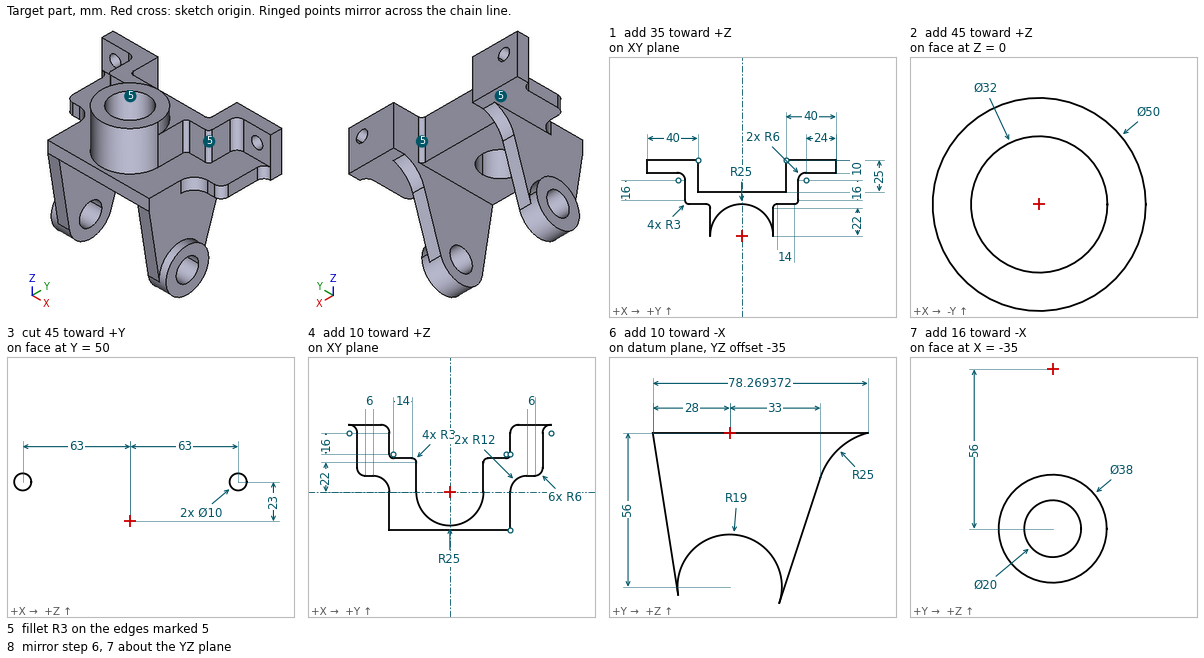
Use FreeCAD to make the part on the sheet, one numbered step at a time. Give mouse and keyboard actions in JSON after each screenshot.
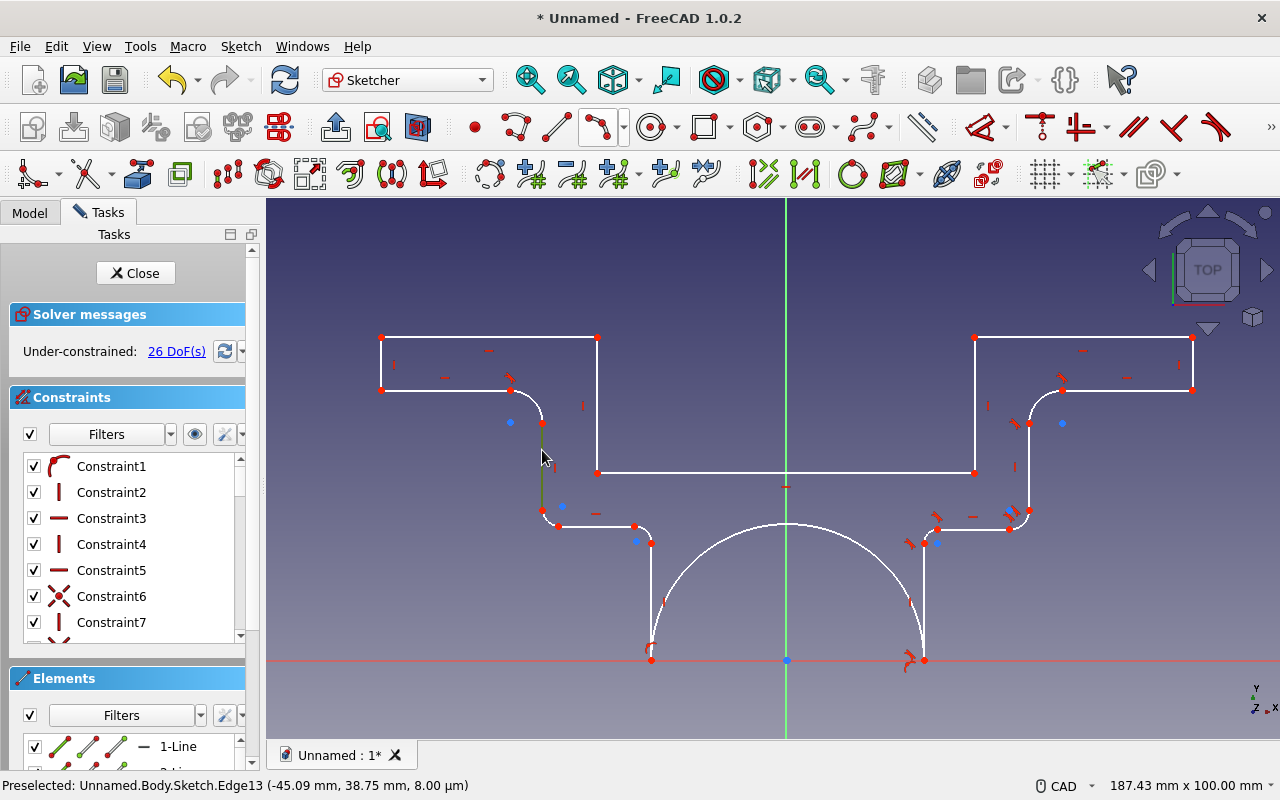
{"action": "left_click", "coordinate": [539, 409]}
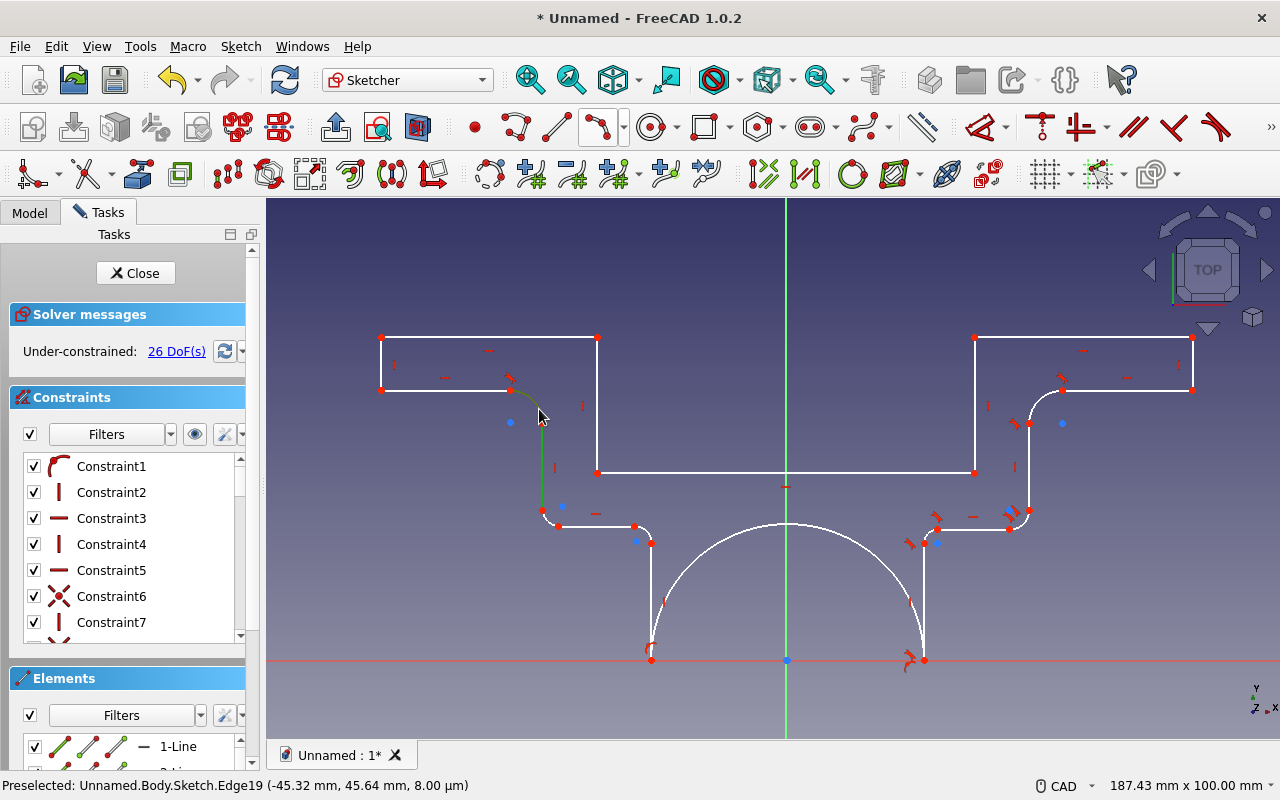
{"action": "left_click", "coordinate": [1216, 128]}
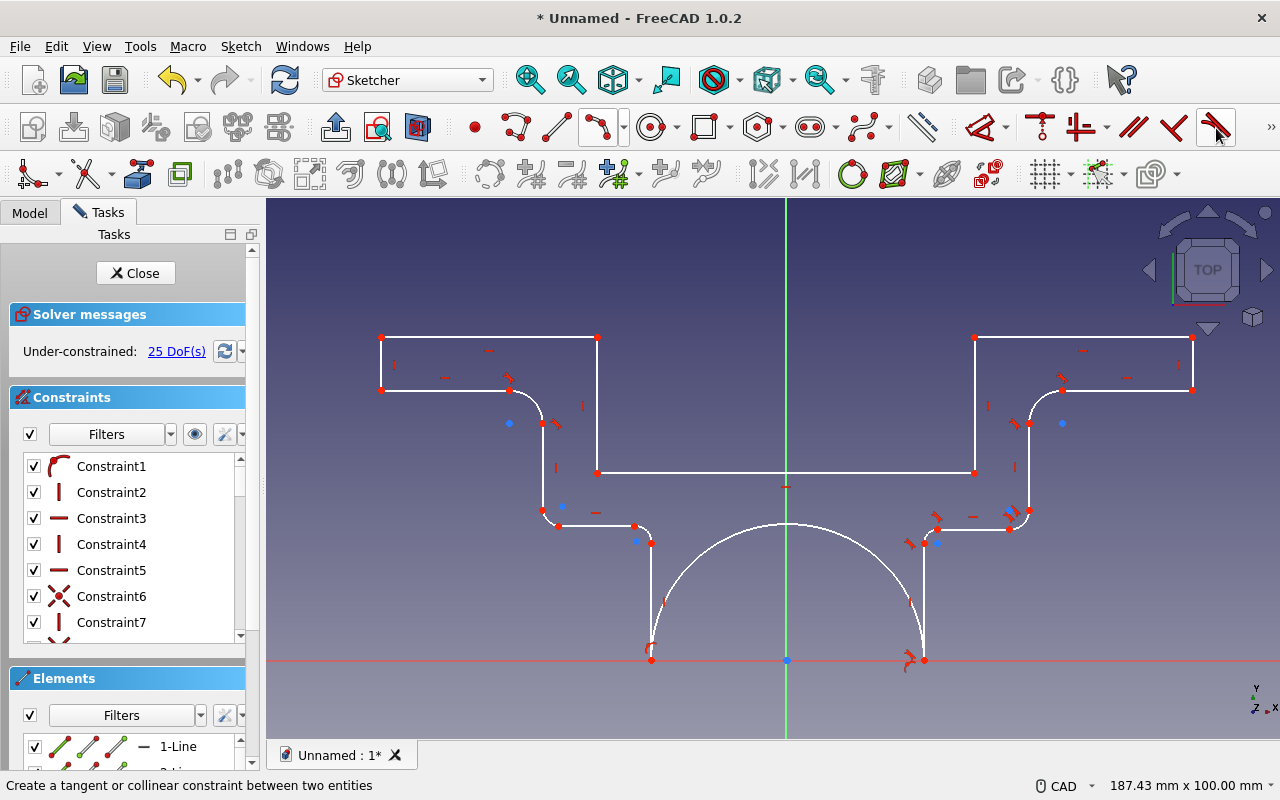
{"action": "left_click", "coordinate": [543, 450]}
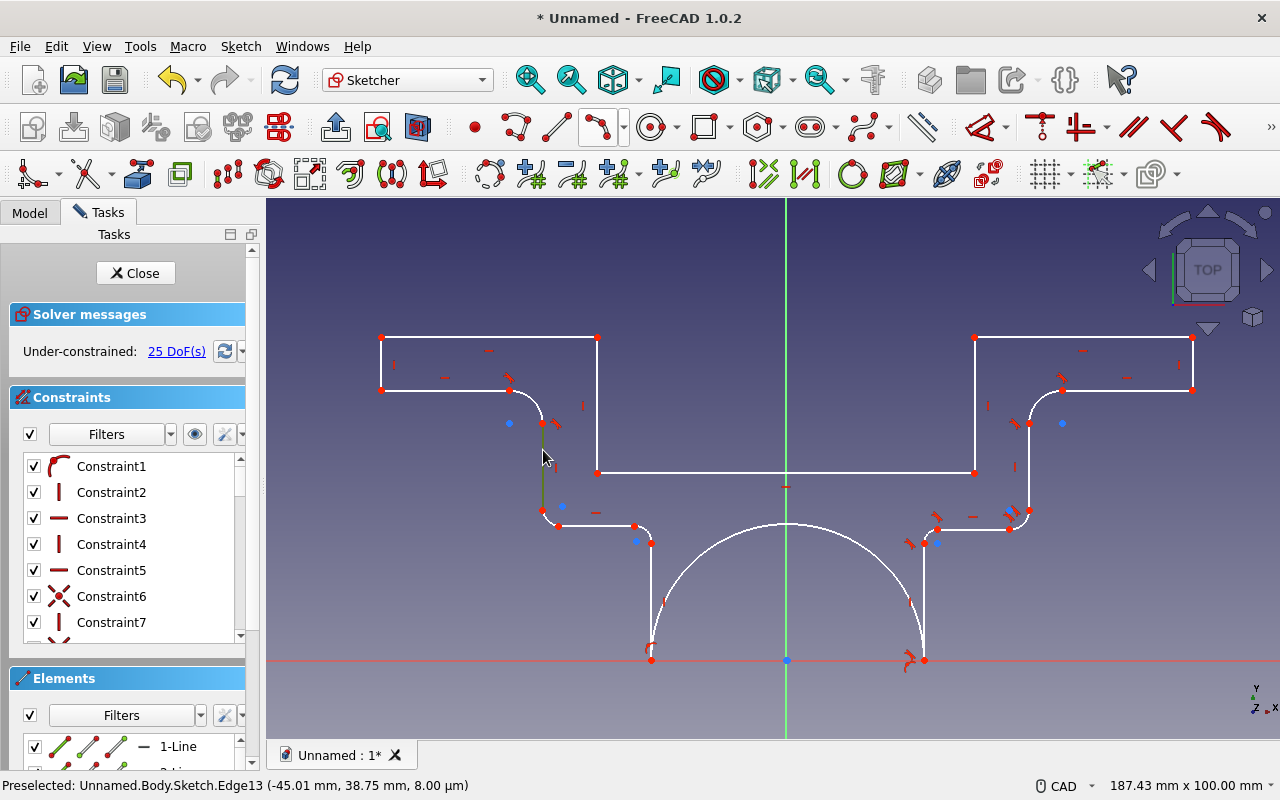
{"action": "left_click", "coordinate": [548, 521]}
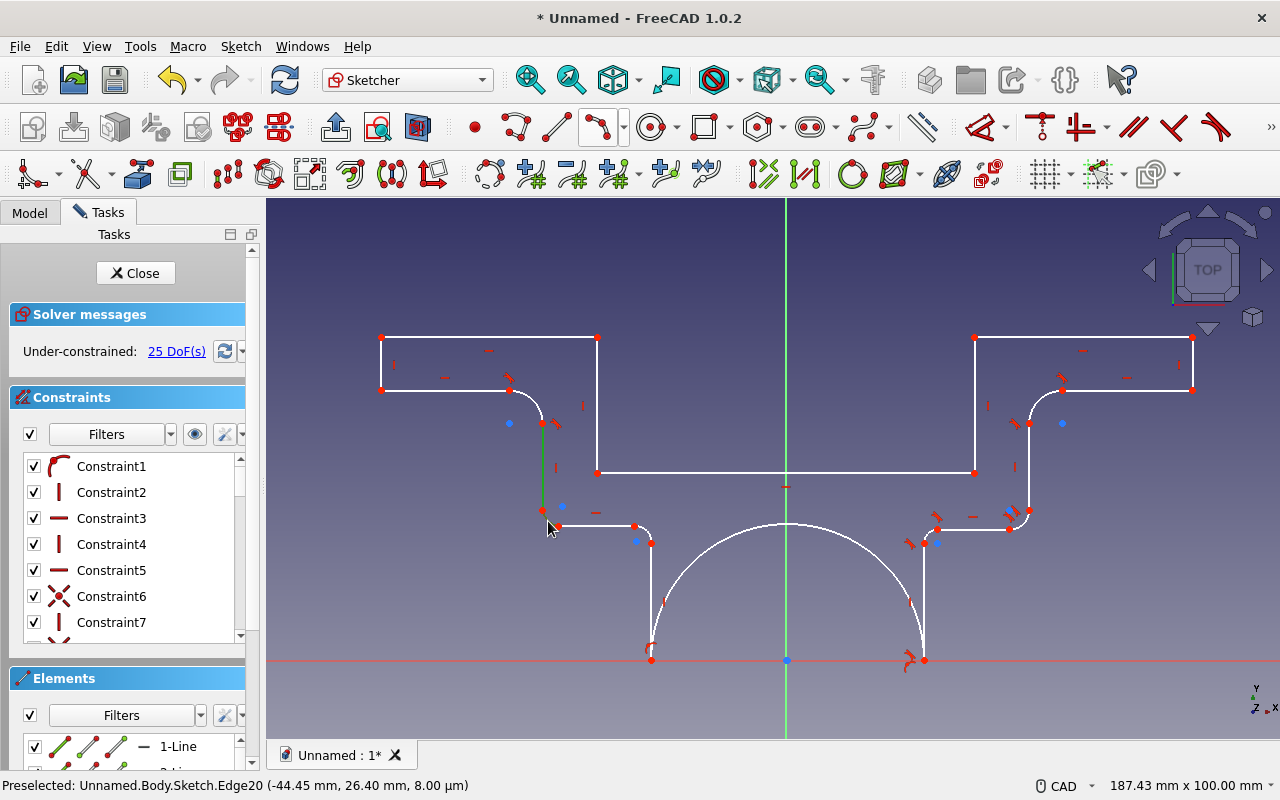
{"action": "left_click", "coordinate": [1216, 128]}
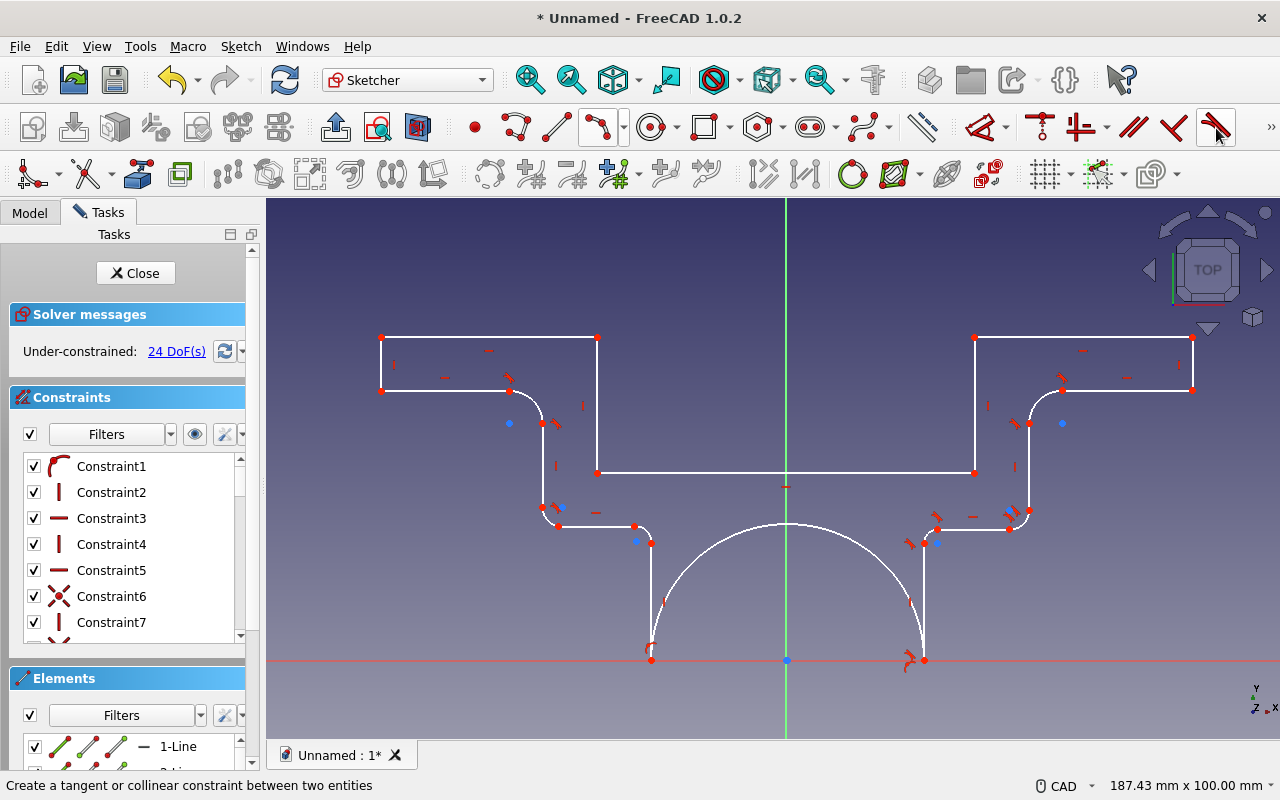
{"action": "left_click", "coordinate": [582, 527]}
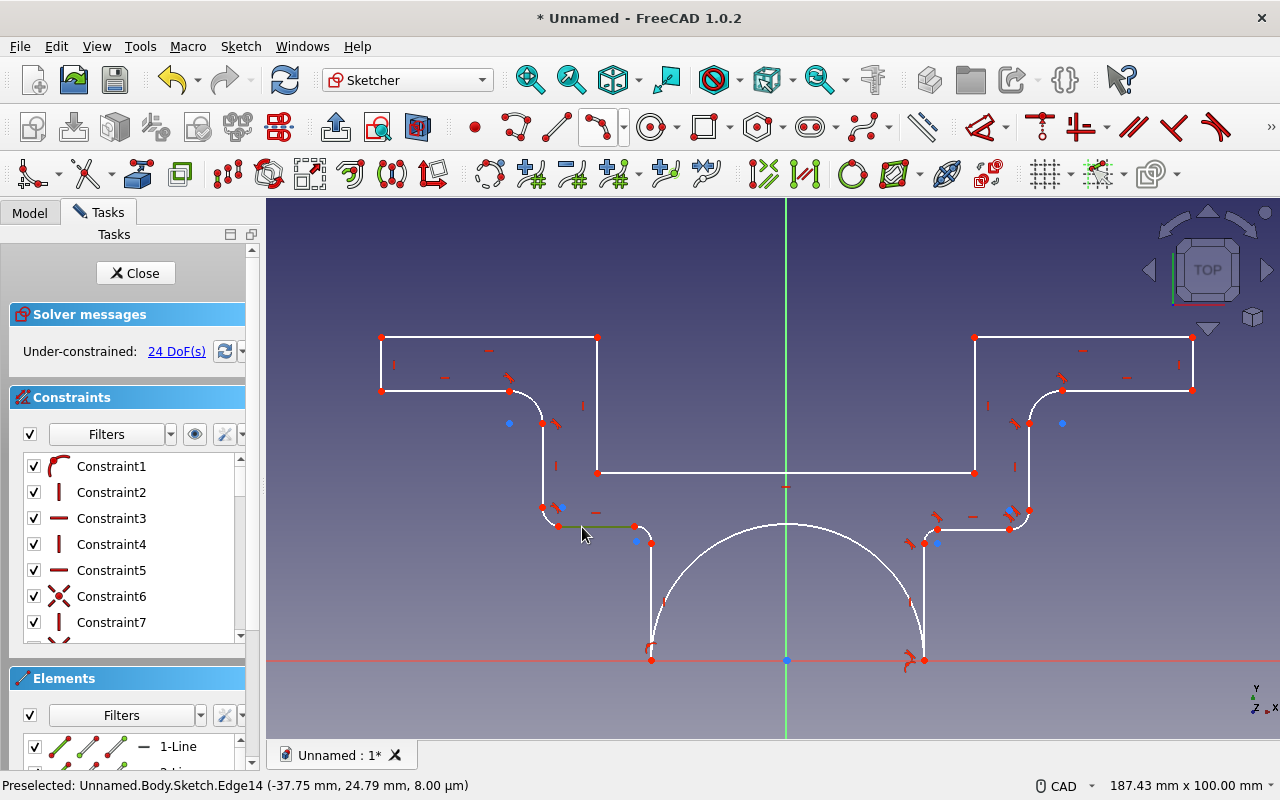
{"action": "left_click", "coordinate": [547, 520]}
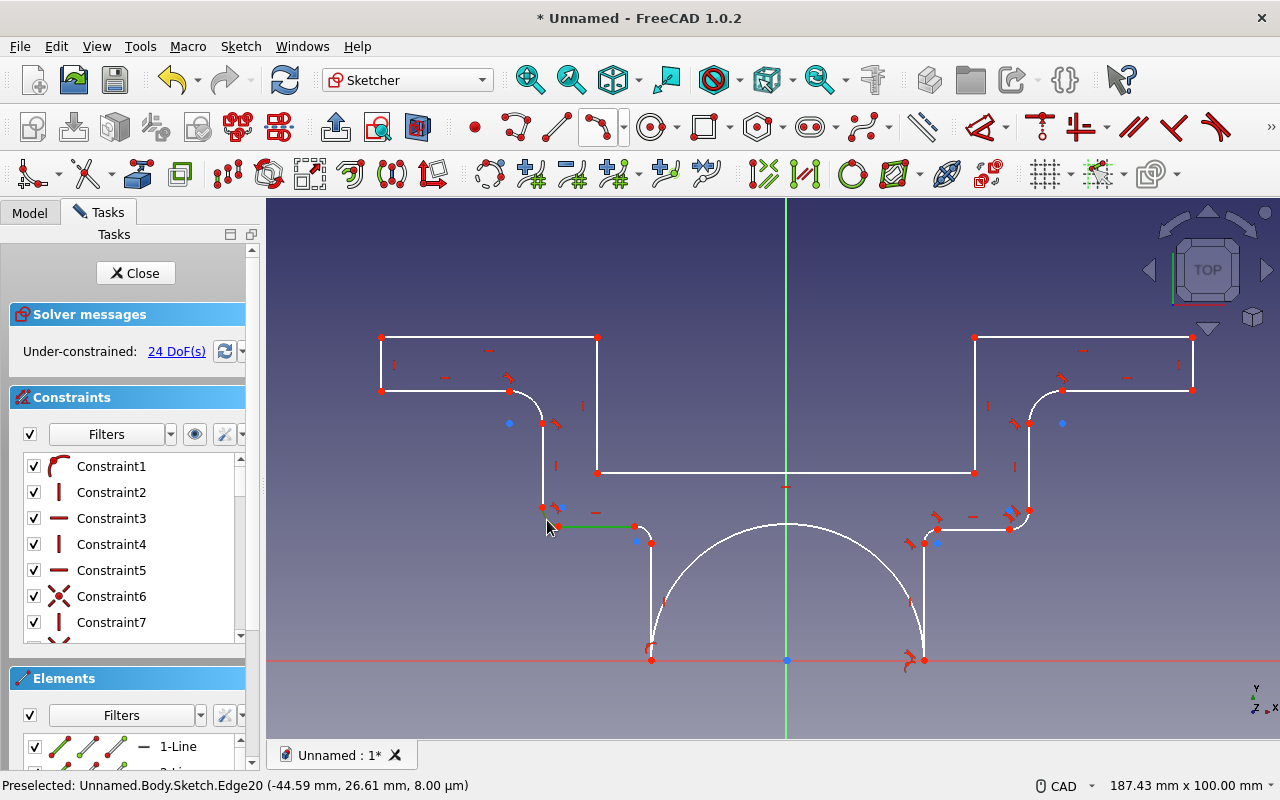
{"action": "left_click", "coordinate": [1216, 128]}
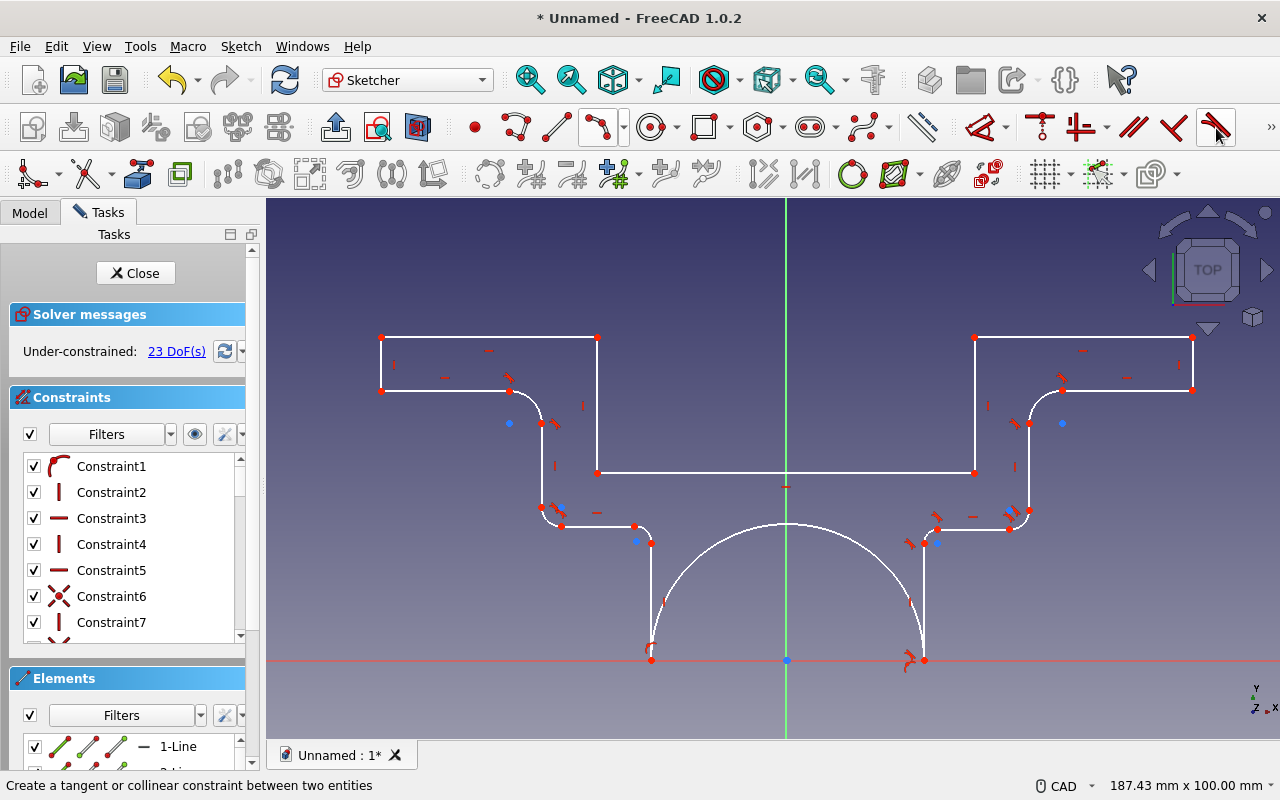
{"action": "left_click", "coordinate": [583, 527]}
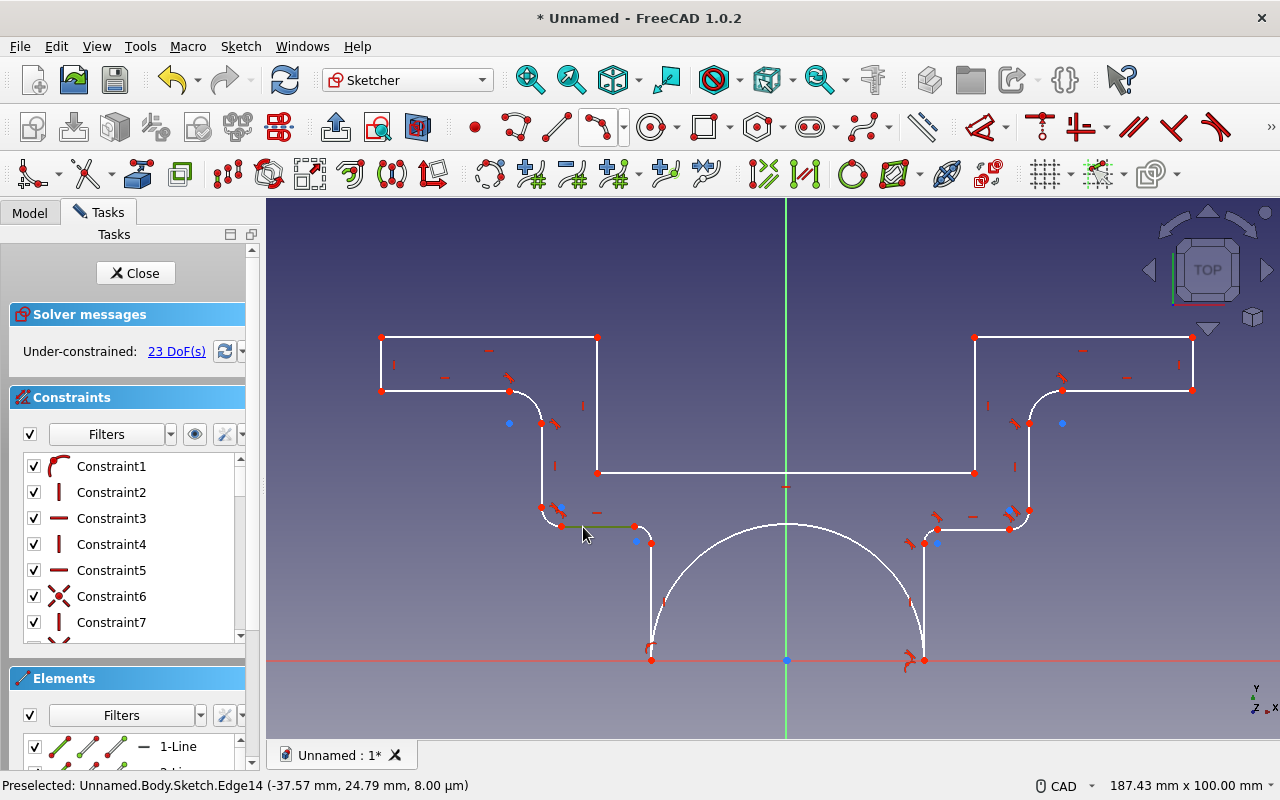
{"action": "left_click", "coordinate": [647, 531]}